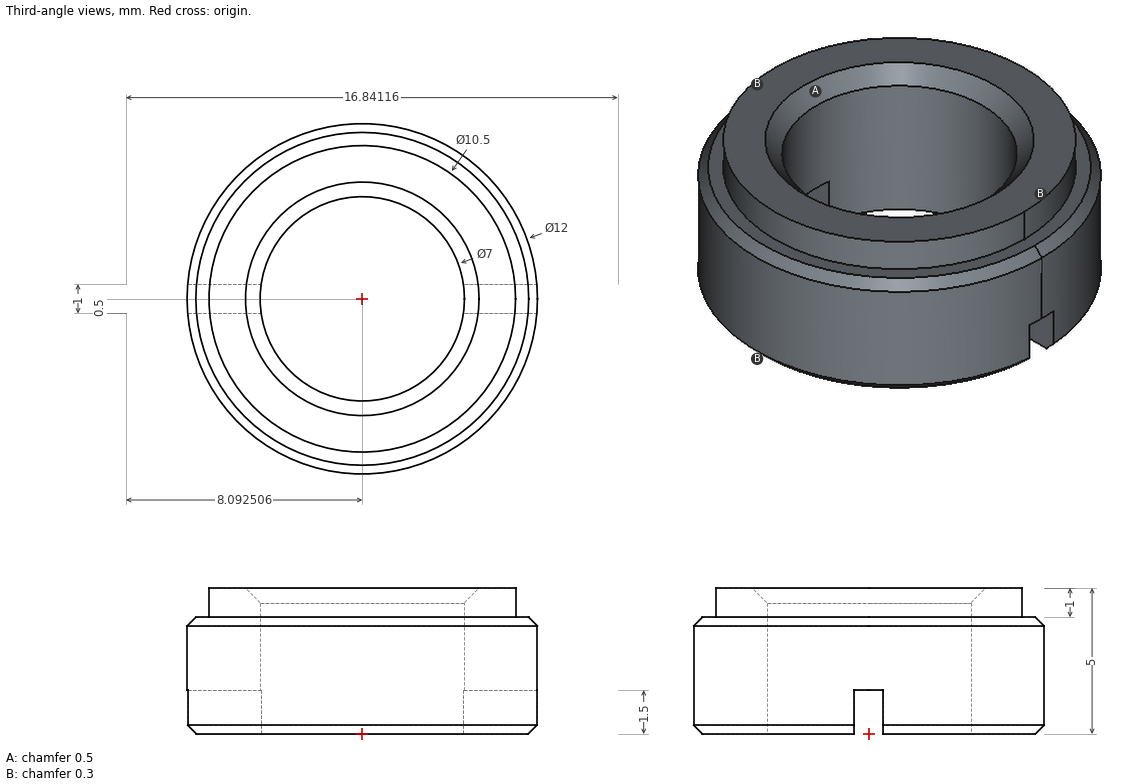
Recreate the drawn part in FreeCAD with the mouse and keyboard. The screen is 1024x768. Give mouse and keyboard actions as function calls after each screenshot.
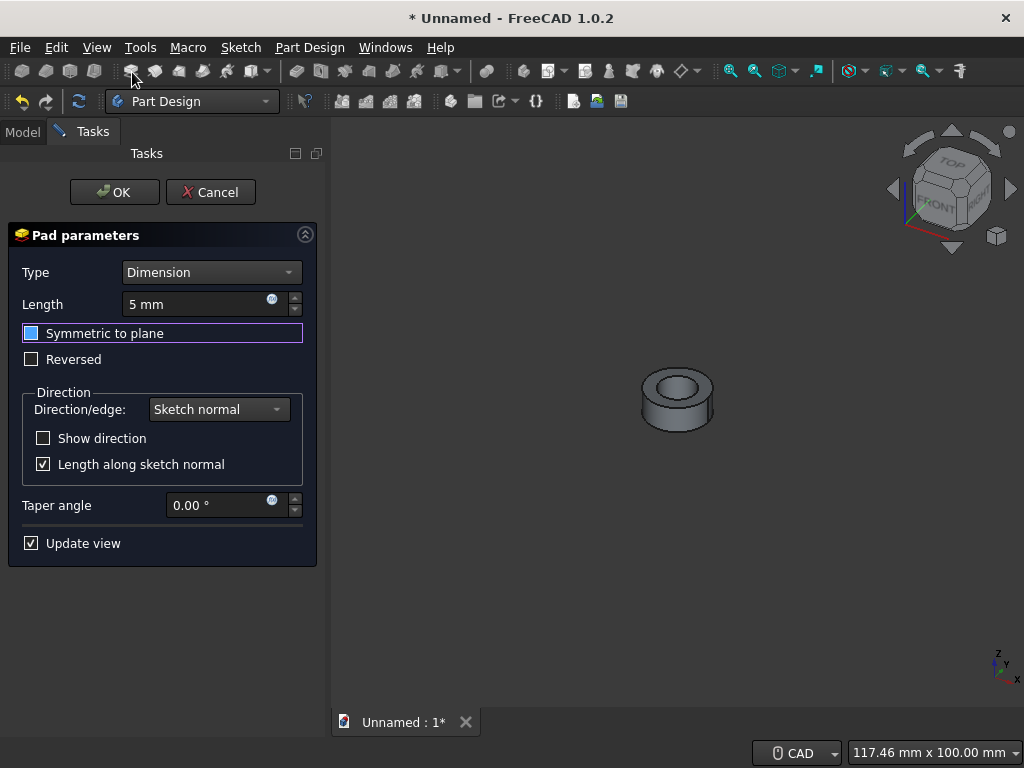
click(115, 192)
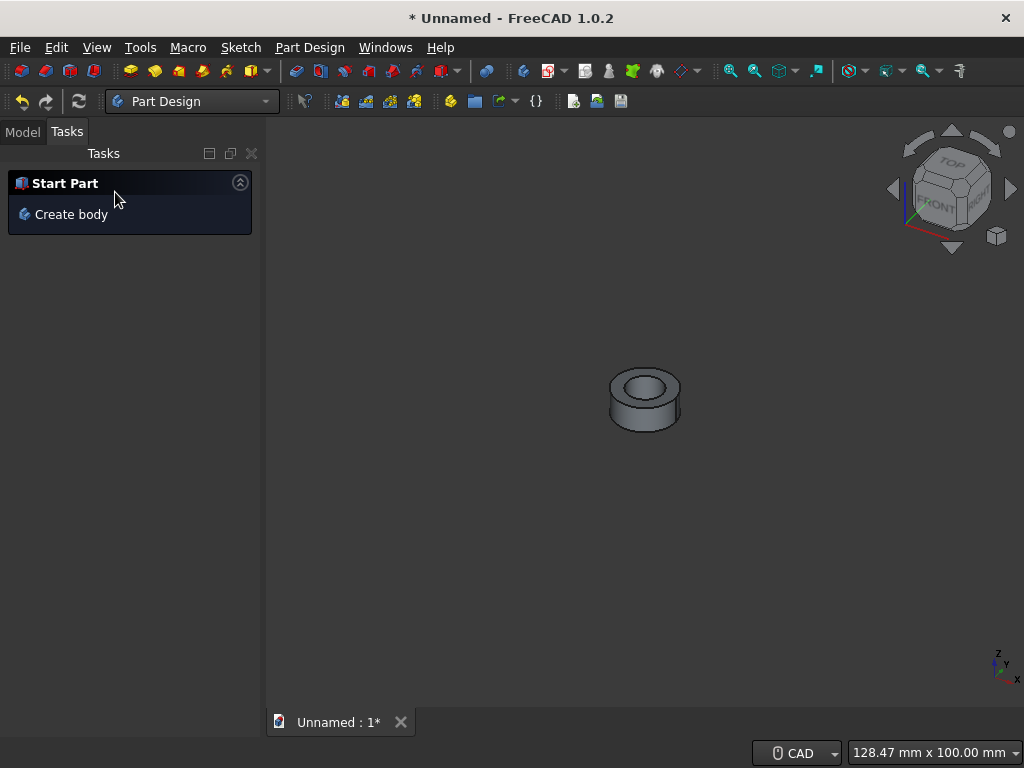
key(v)
key(f)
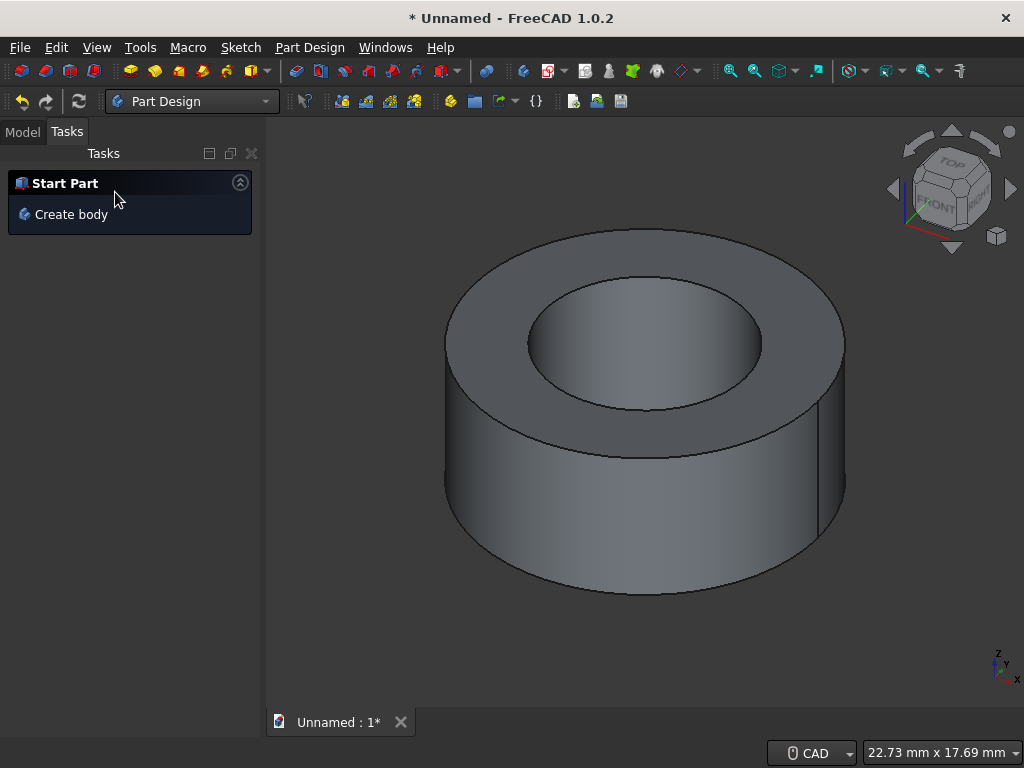
click(544, 309)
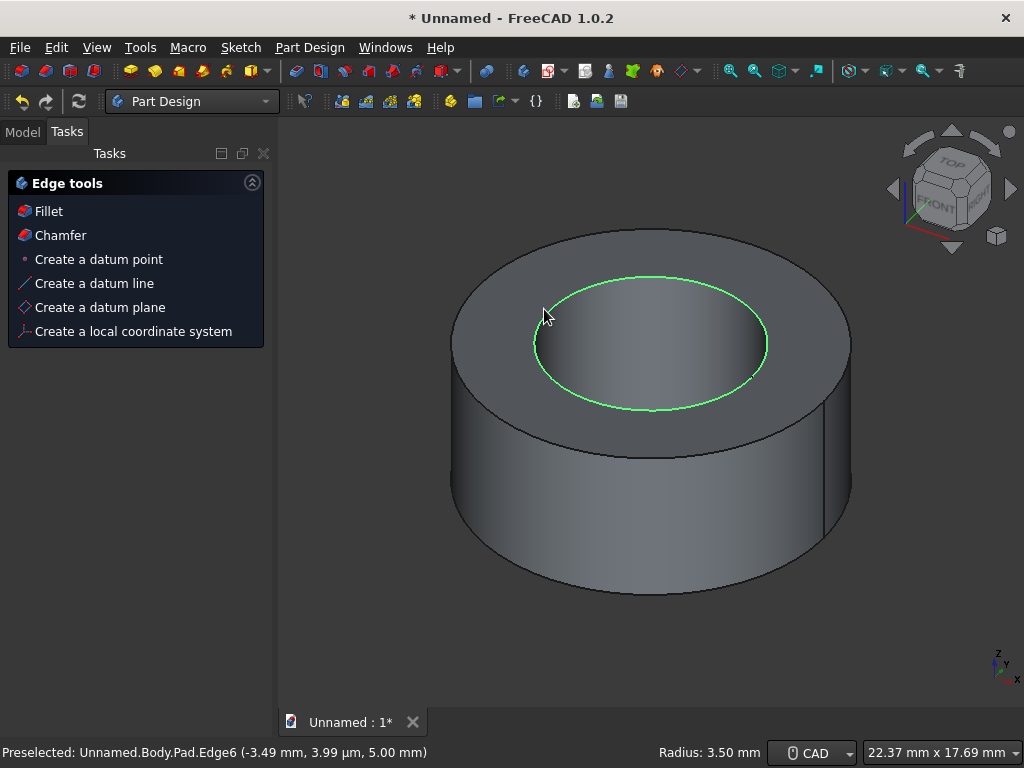
click(46, 72)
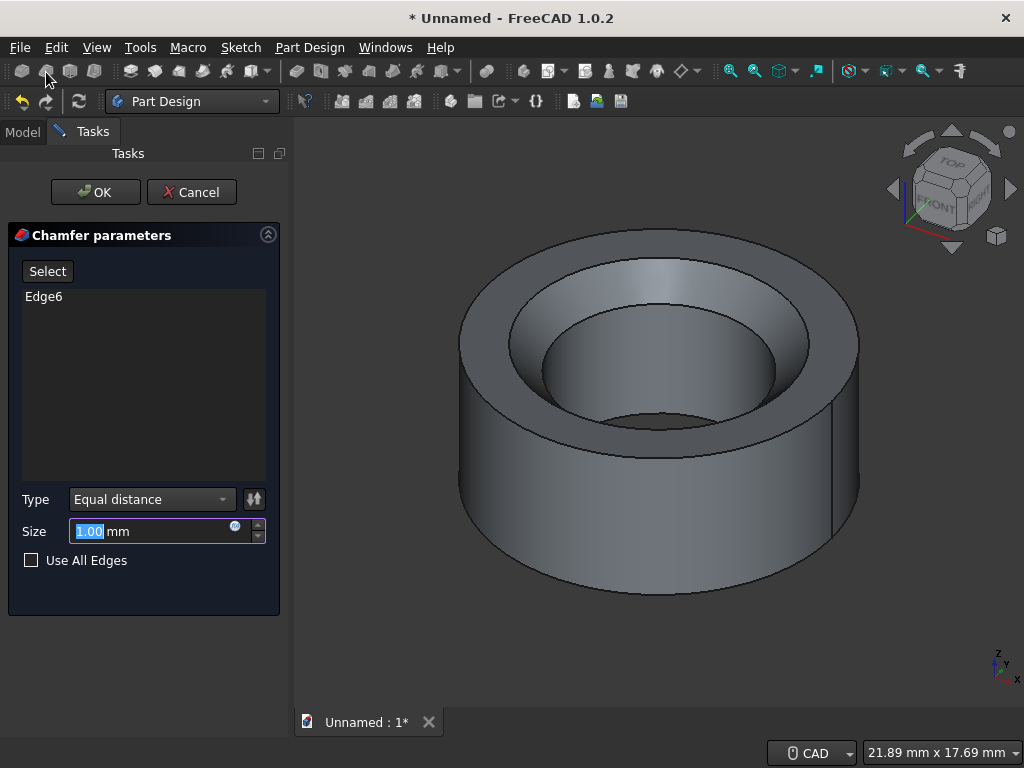
text(0.5)
key(Tab)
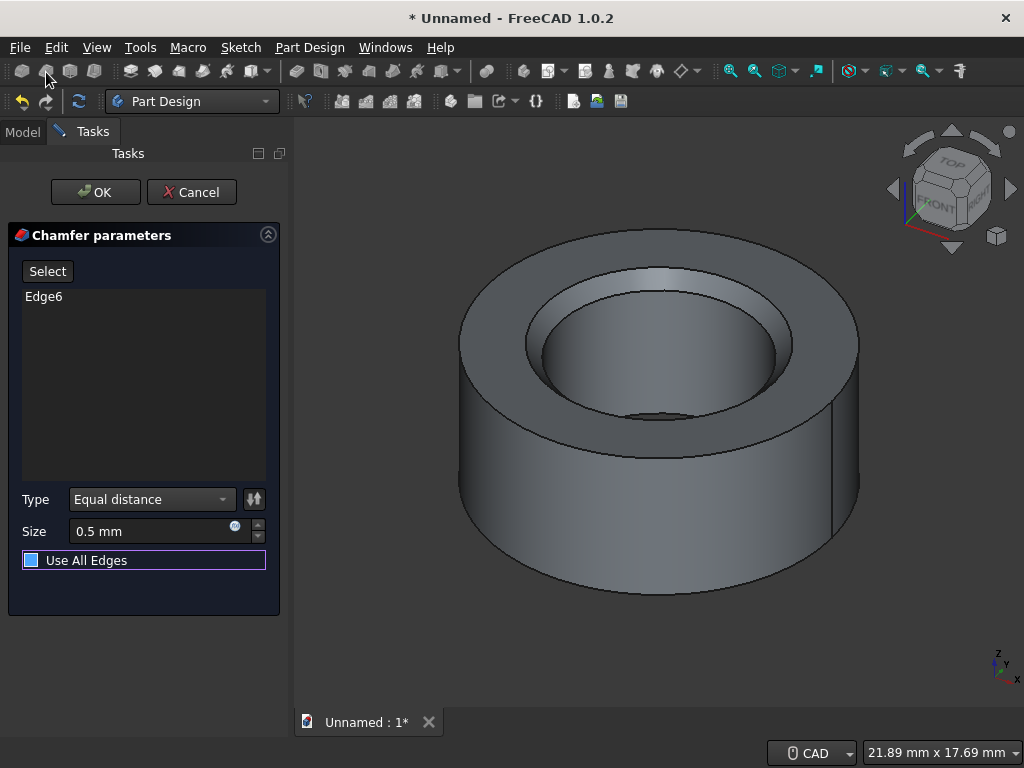
click(96, 192)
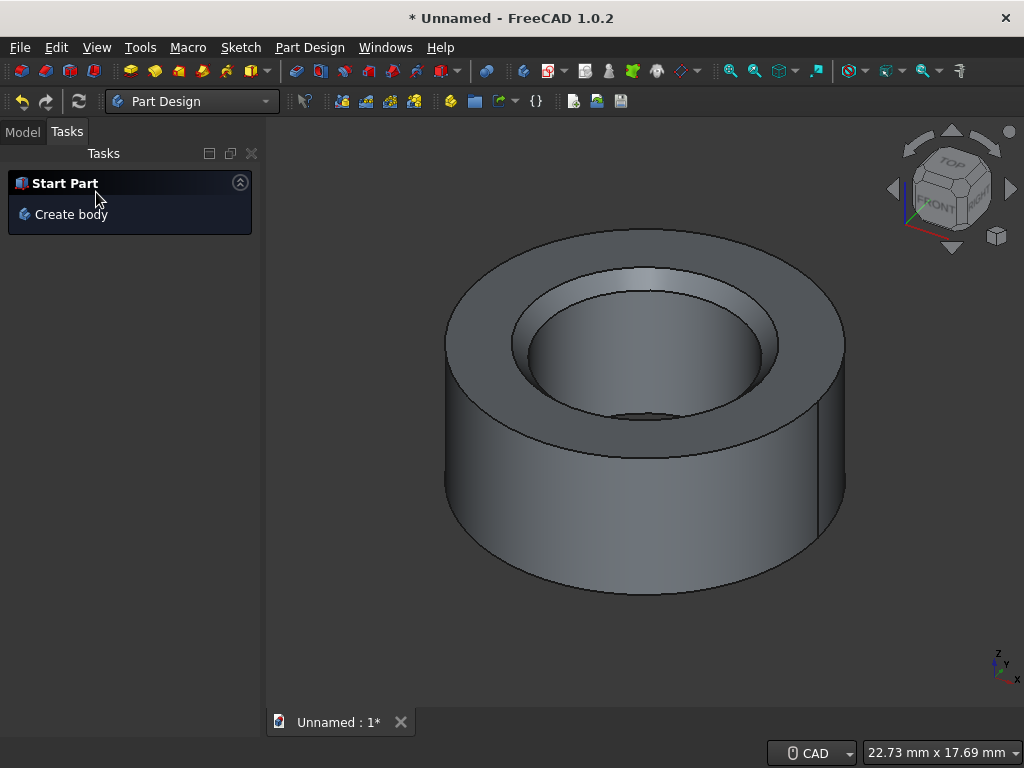
key(5)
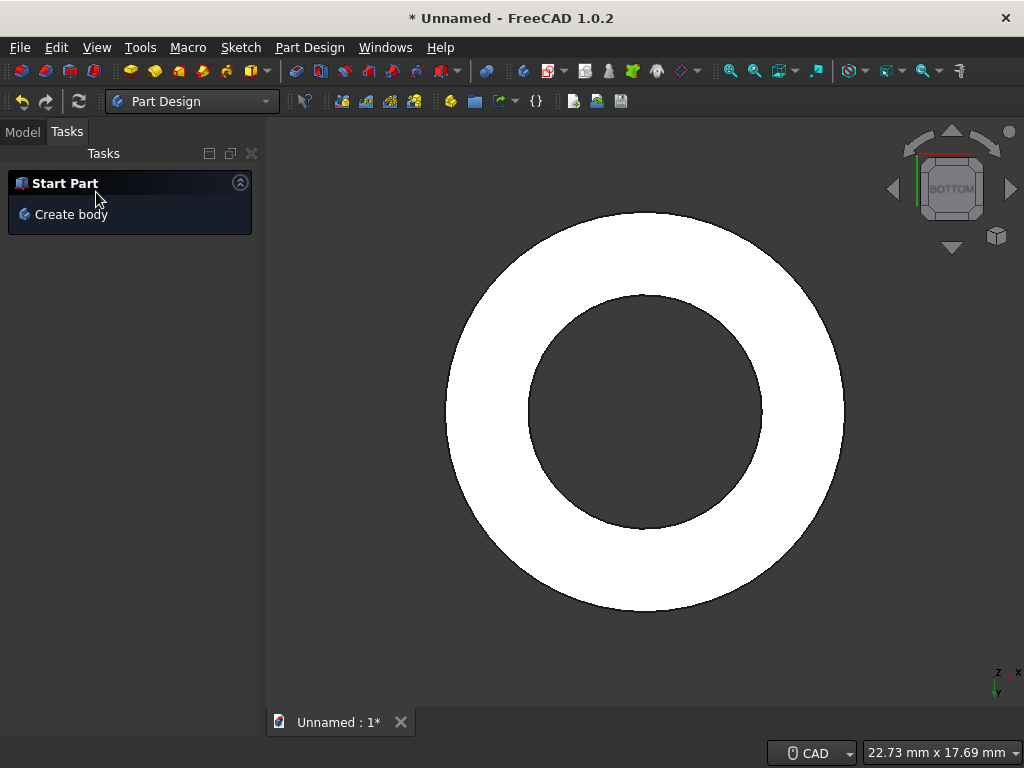
click(759, 525)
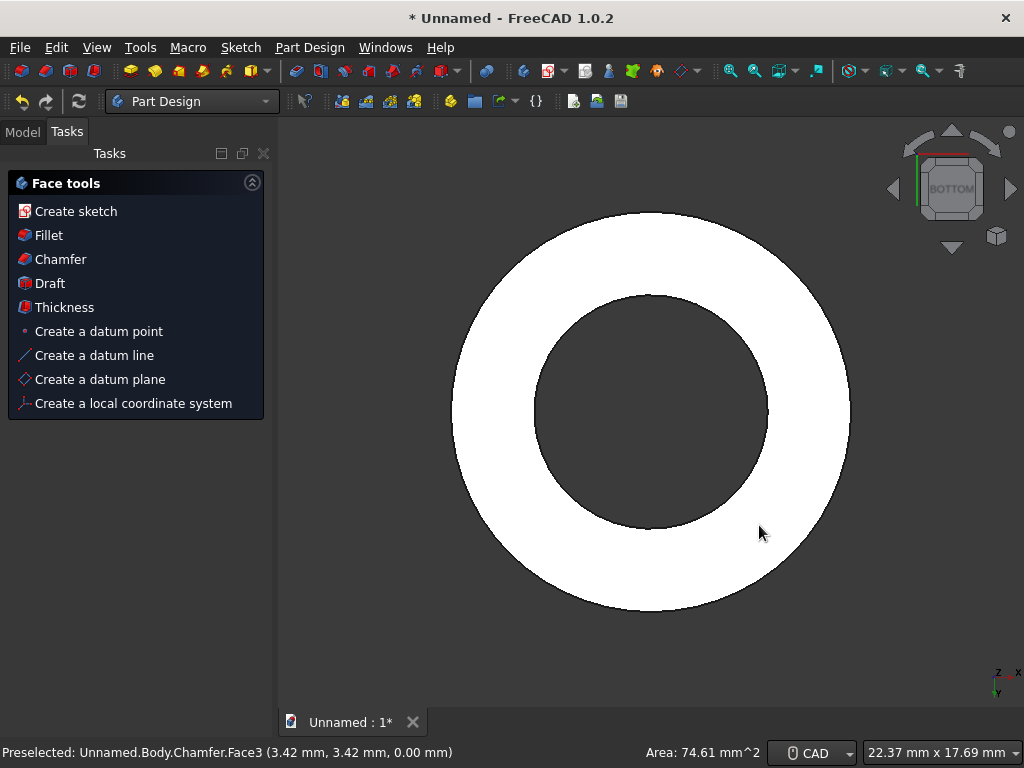
click(548, 72)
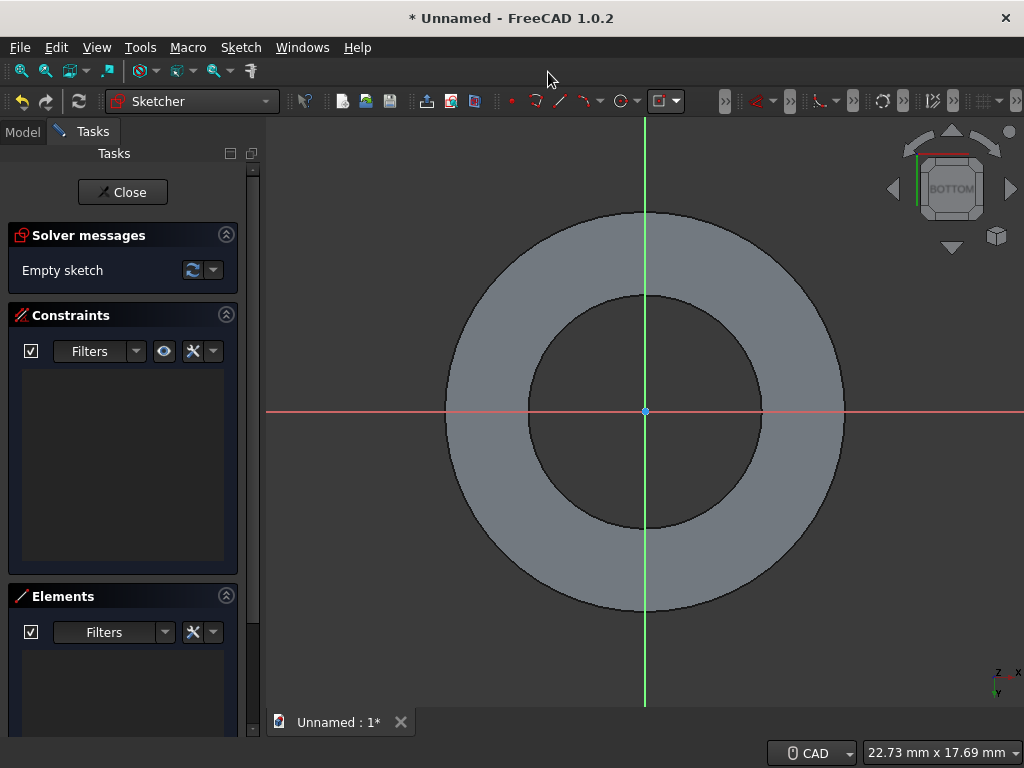
scroll(415, 412, down, 2)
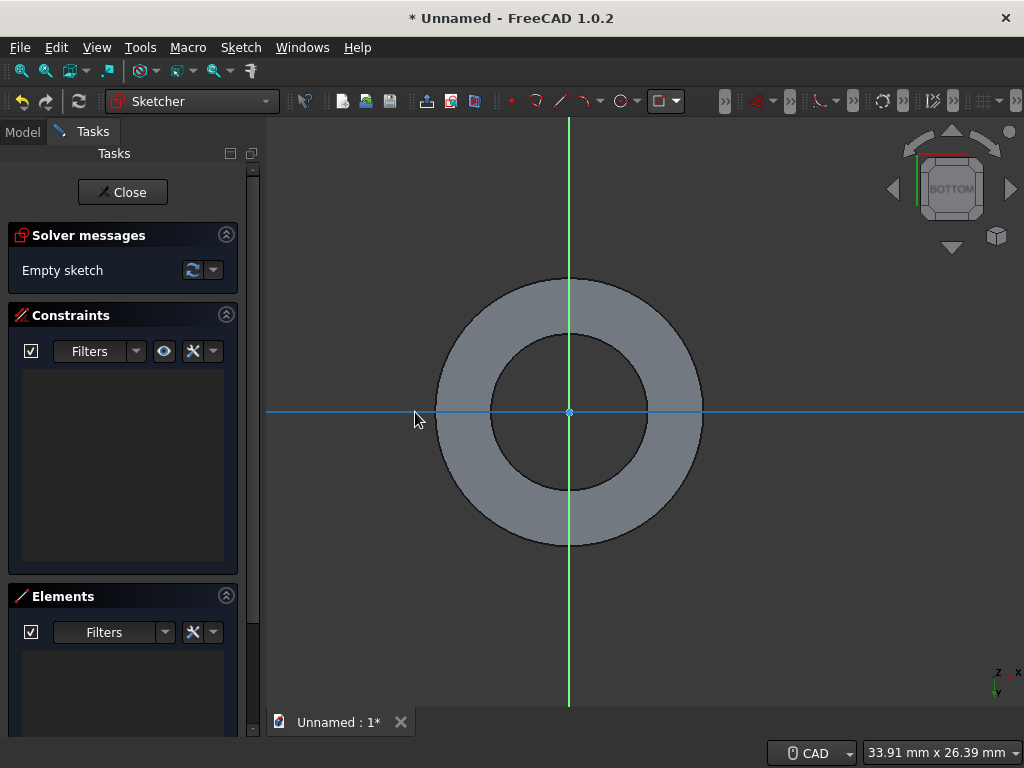
click(678, 102)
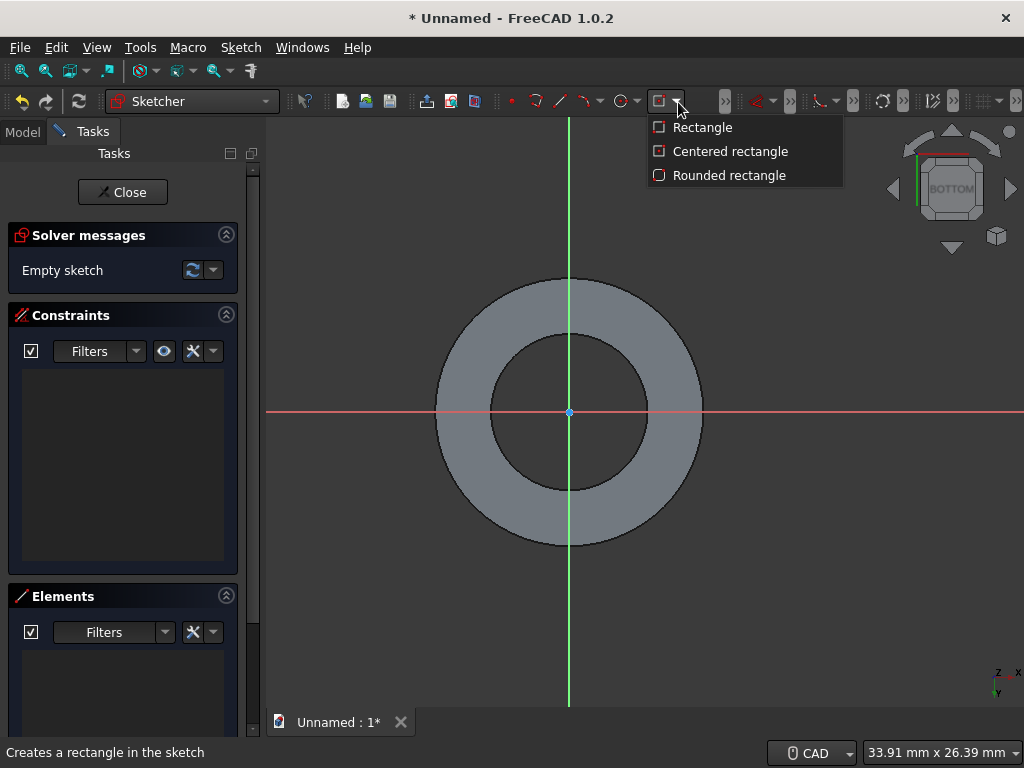
click(746, 127)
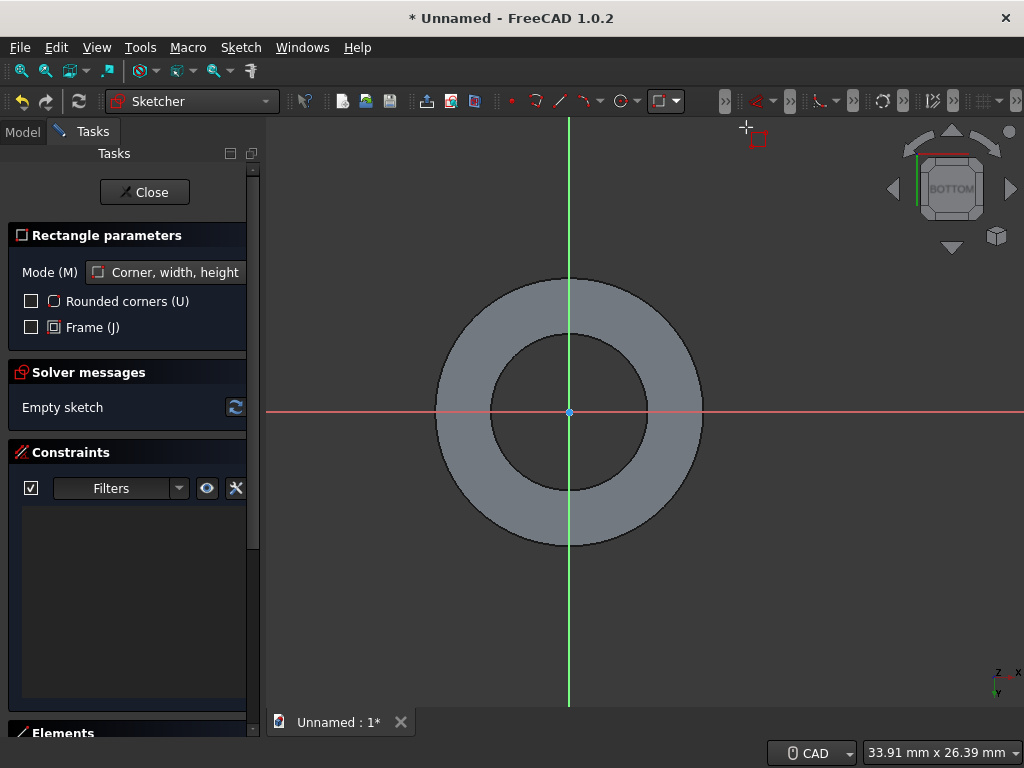
scroll(388, 401, up, 2)